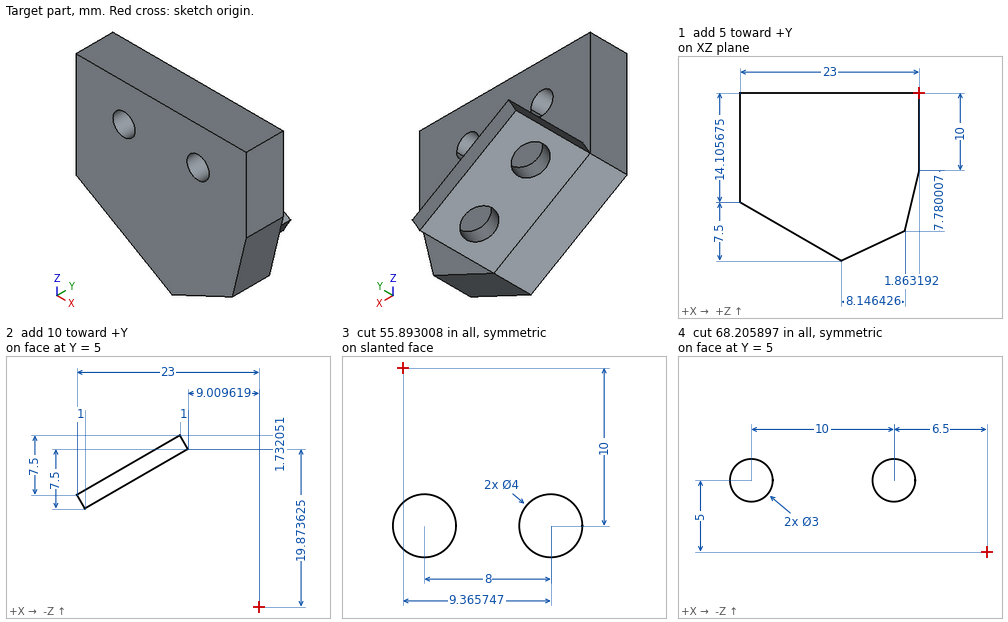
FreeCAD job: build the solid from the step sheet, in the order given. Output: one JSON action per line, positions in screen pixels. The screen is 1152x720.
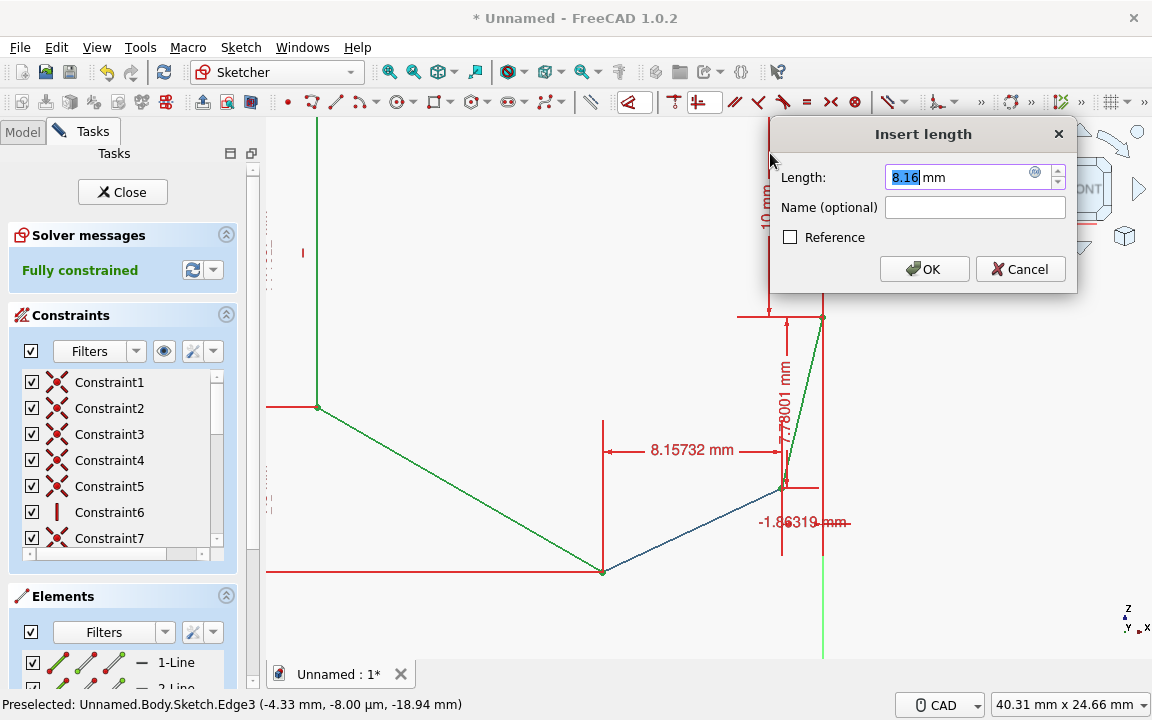
{"action": "type", "text": "8.146426"}
{"action": "key", "text": "Return"}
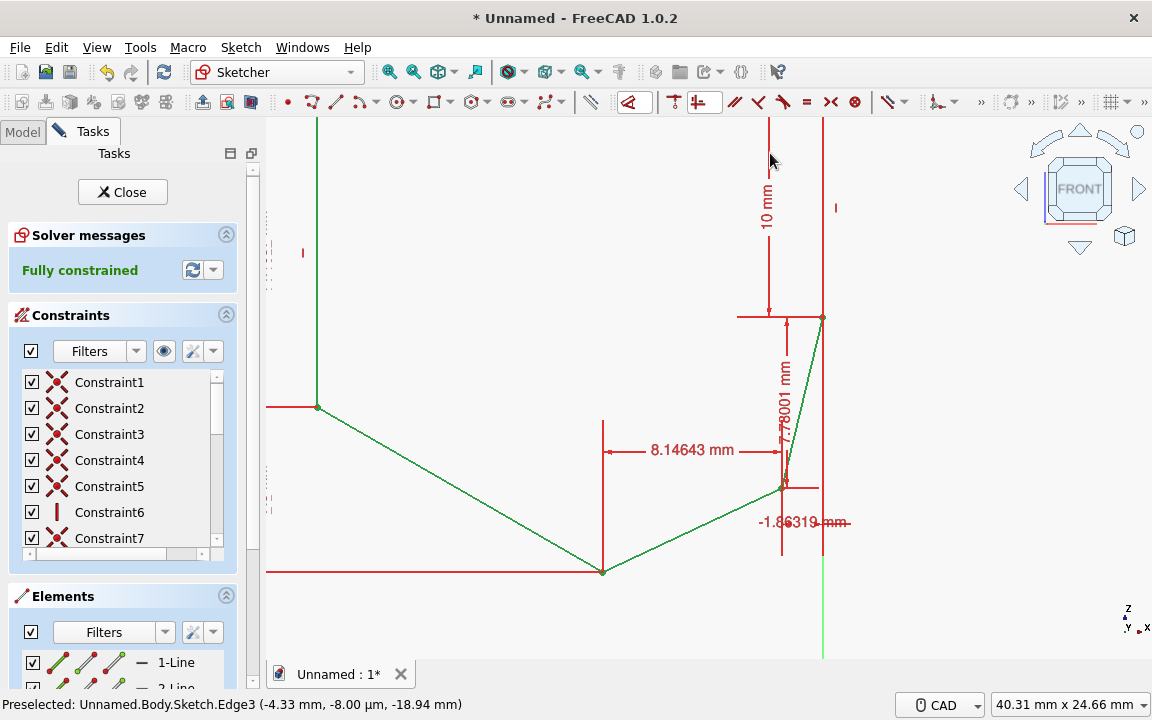
{"action": "left_click", "coordinate": [123, 192]}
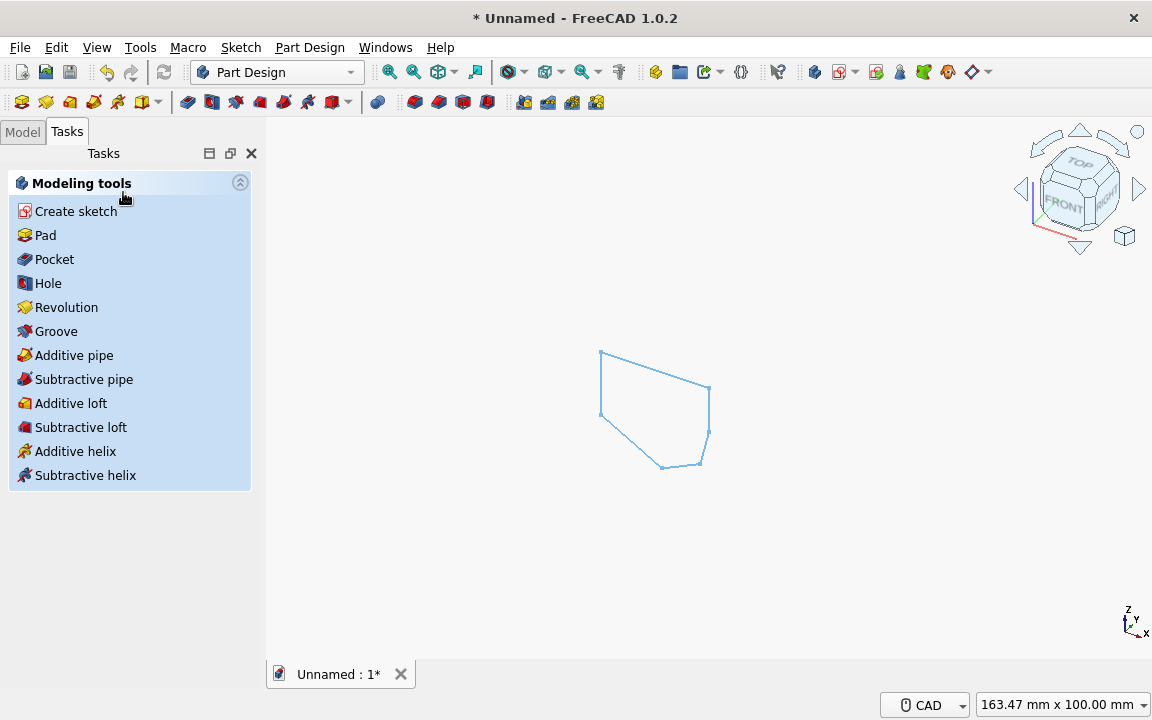
{"action": "left_click", "coordinate": [22, 102]}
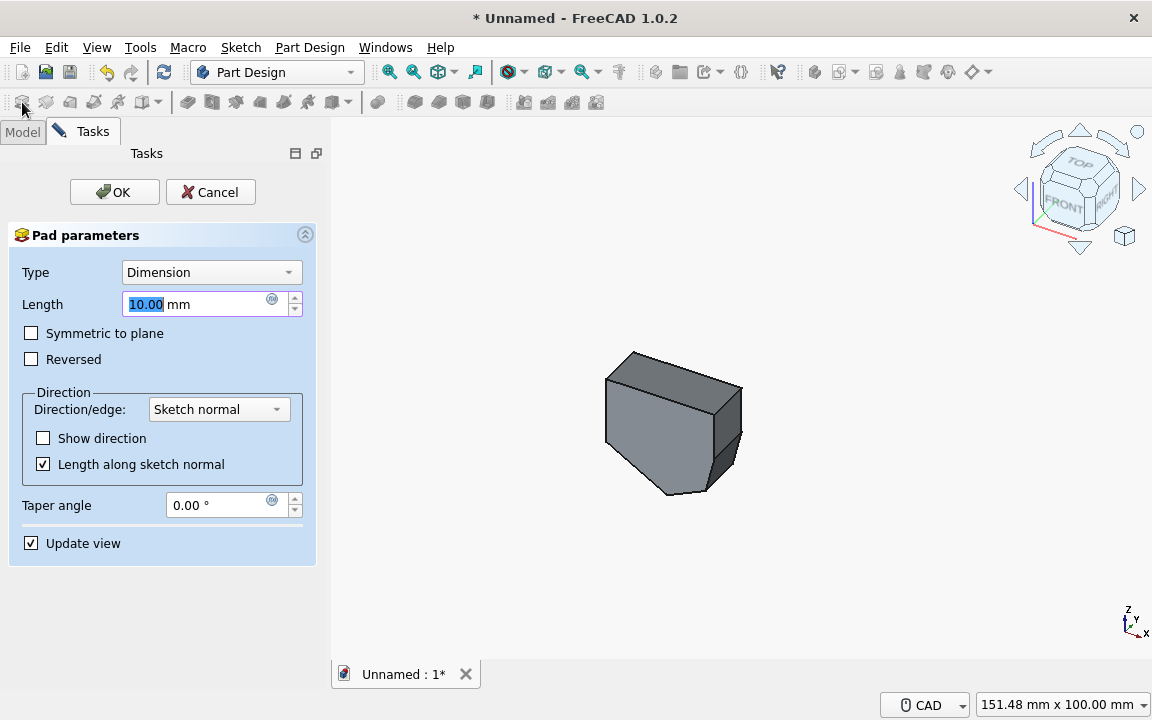
{"action": "type", "text": "5"}
{"action": "key", "text": "Tab"}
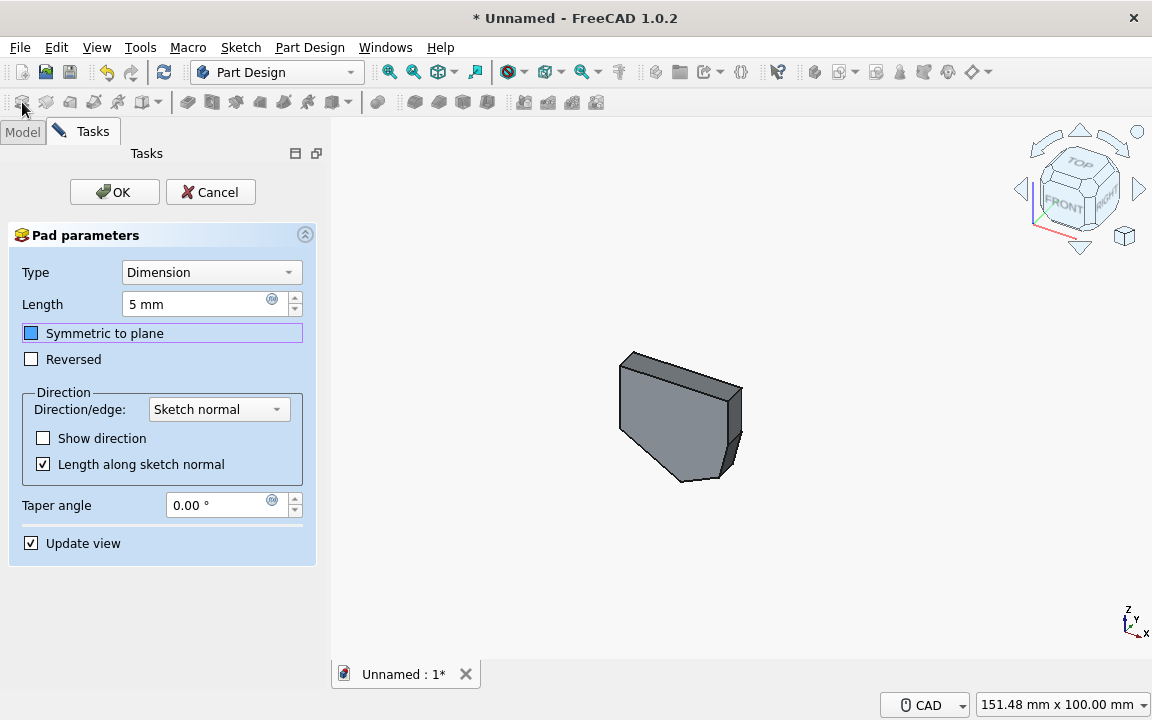
{"action": "left_click", "coordinate": [30, 359]}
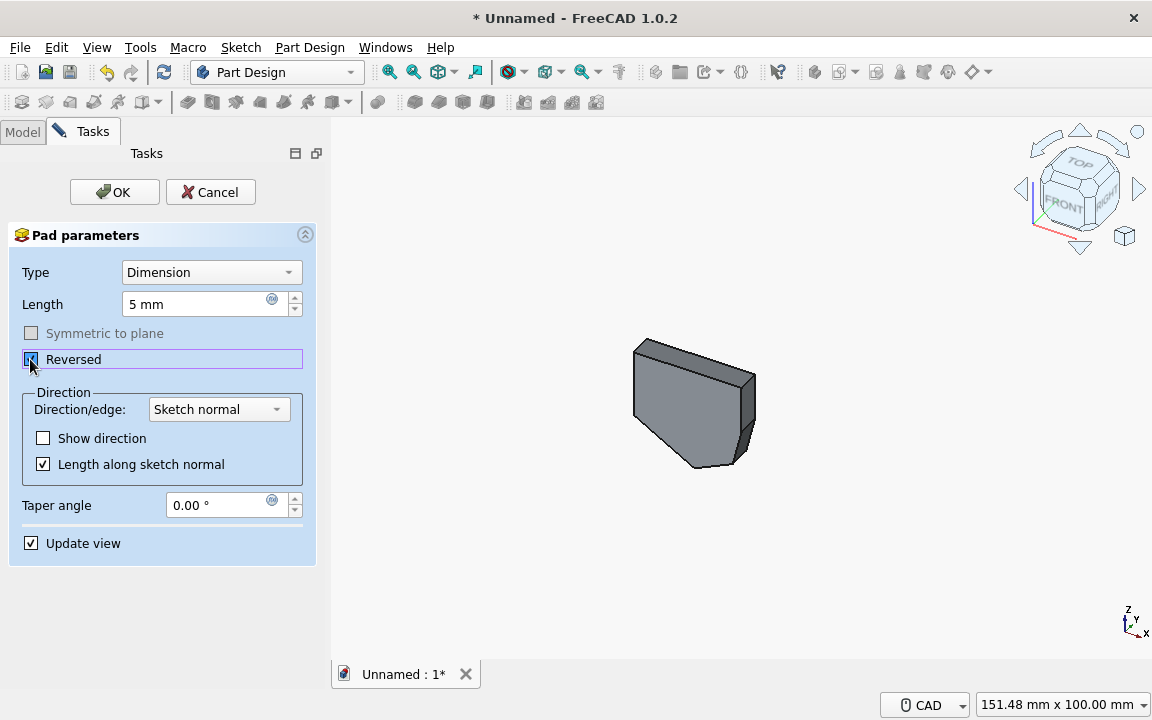
{"action": "left_click", "coordinate": [115, 192]}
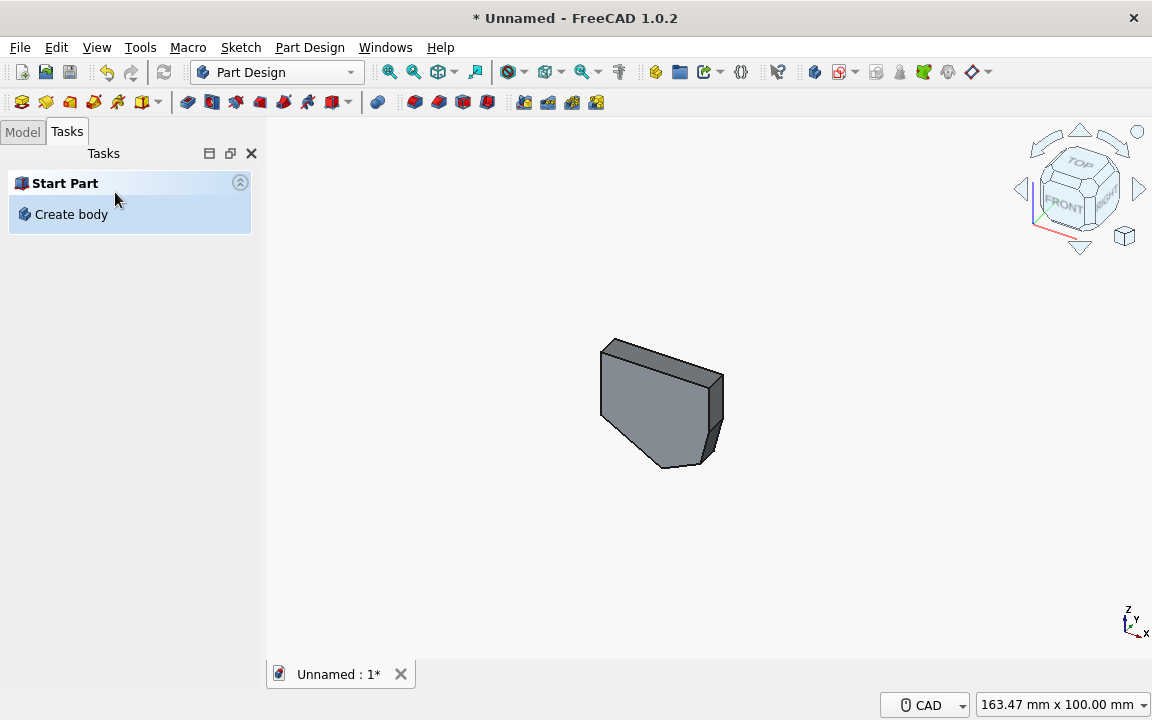
{"action": "left_click", "coordinate": [390, 72]}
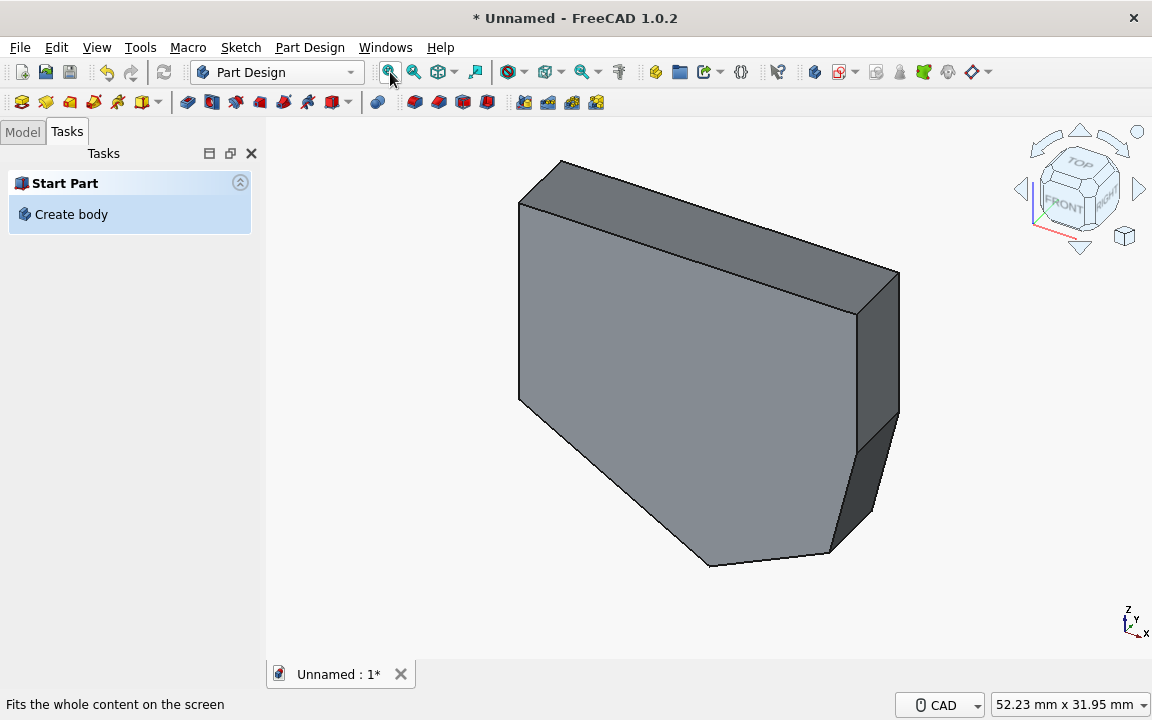
{"action": "key", "text": "4"}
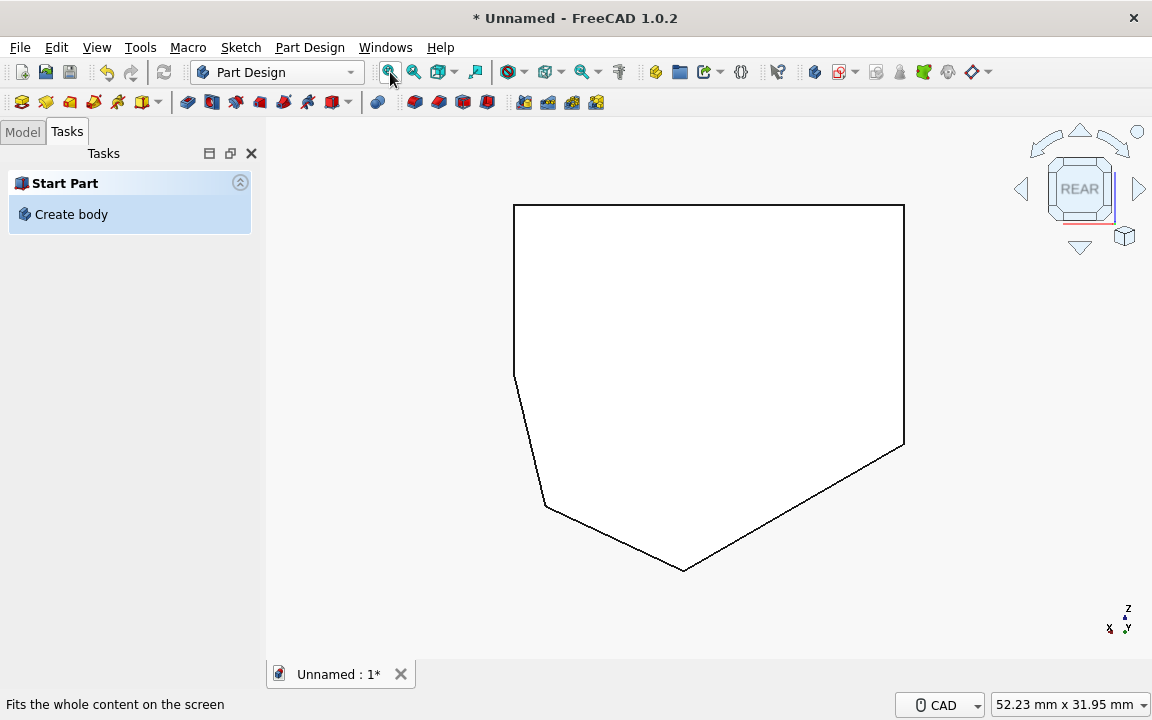
{"action": "left_click", "coordinate": [709, 387]}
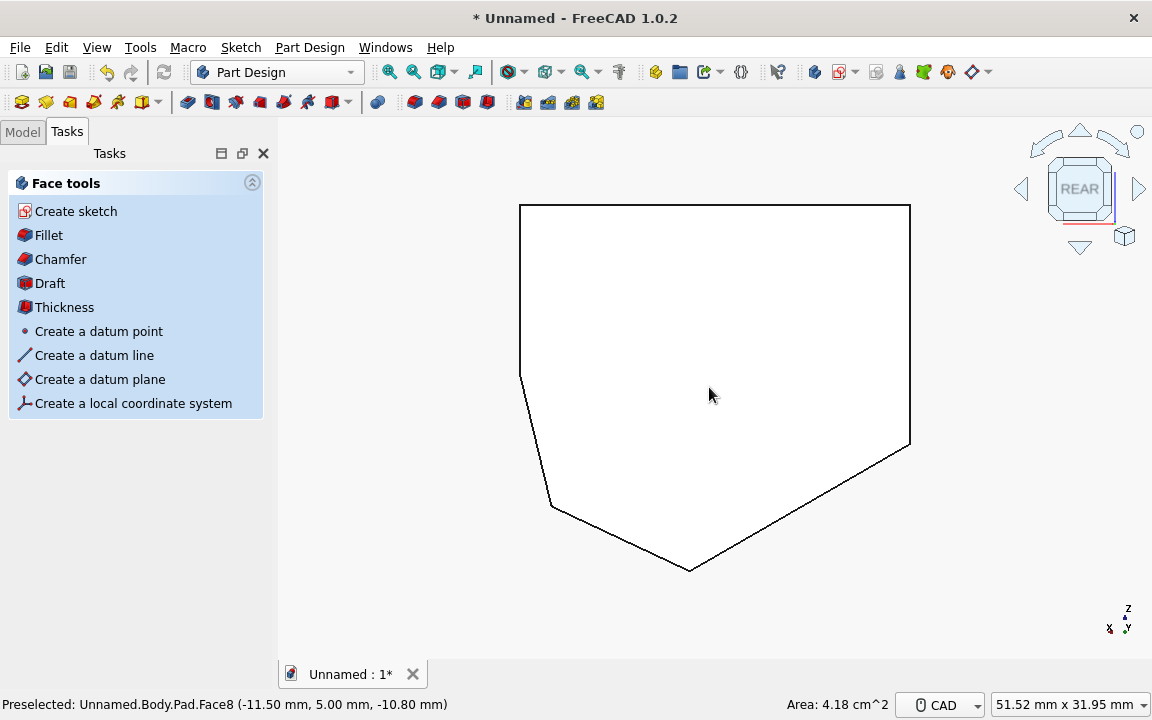
{"action": "left_click", "coordinate": [840, 72]}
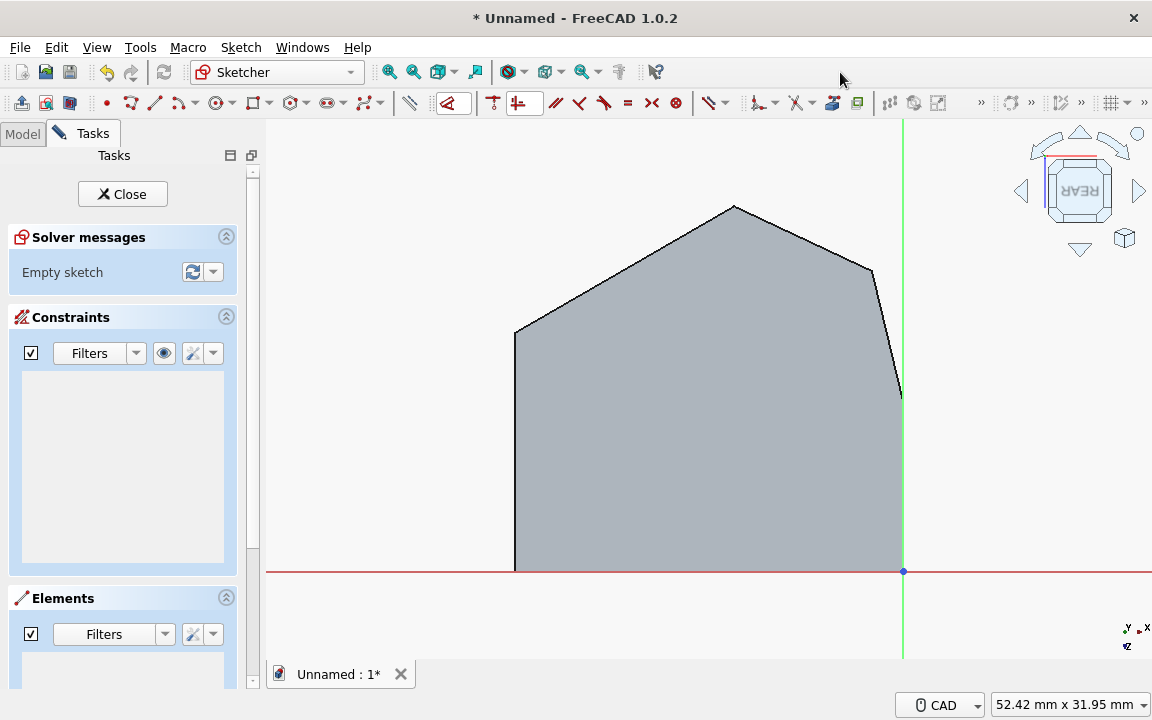
{"action": "left_click", "coordinate": [132, 104]}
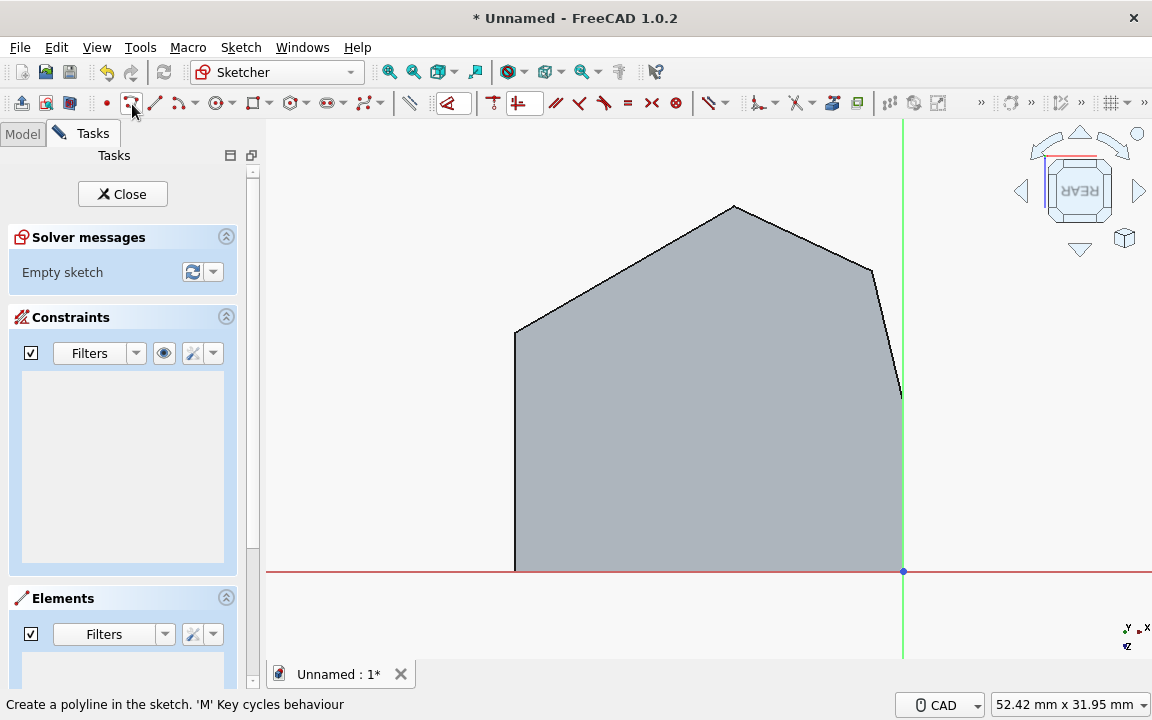
{"action": "left_click", "coordinate": [751, 236]}
{"action": "left_click", "coordinate": [734, 206]}
{"action": "left_click", "coordinate": [515, 333]}
{"action": "left_click", "coordinate": [532, 362]}
{"action": "left_click", "coordinate": [751, 237]}
{"action": "key", "text": "Escape"}
{"action": "key", "text": "Escape"}